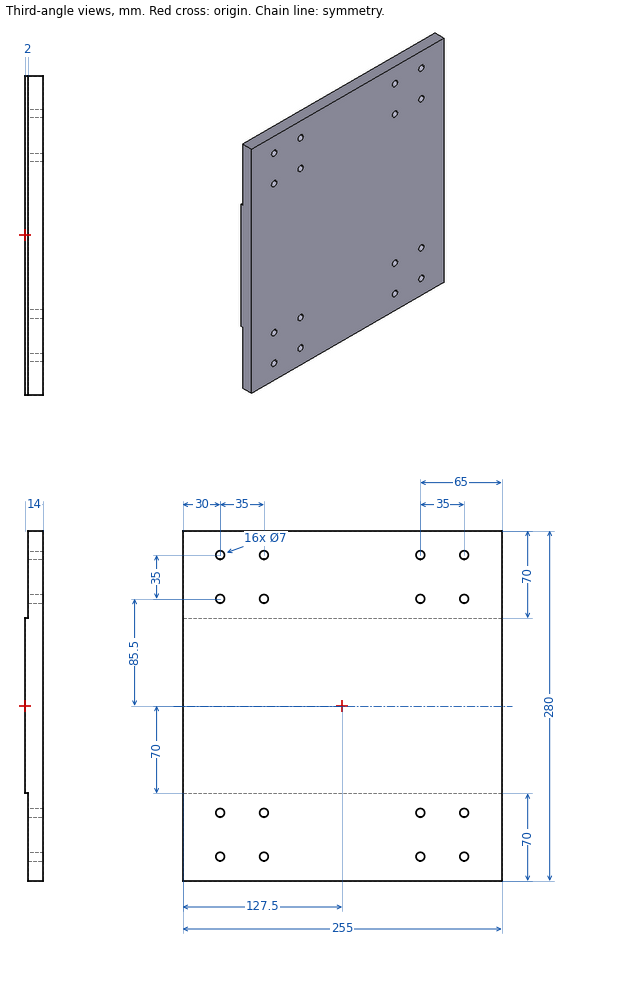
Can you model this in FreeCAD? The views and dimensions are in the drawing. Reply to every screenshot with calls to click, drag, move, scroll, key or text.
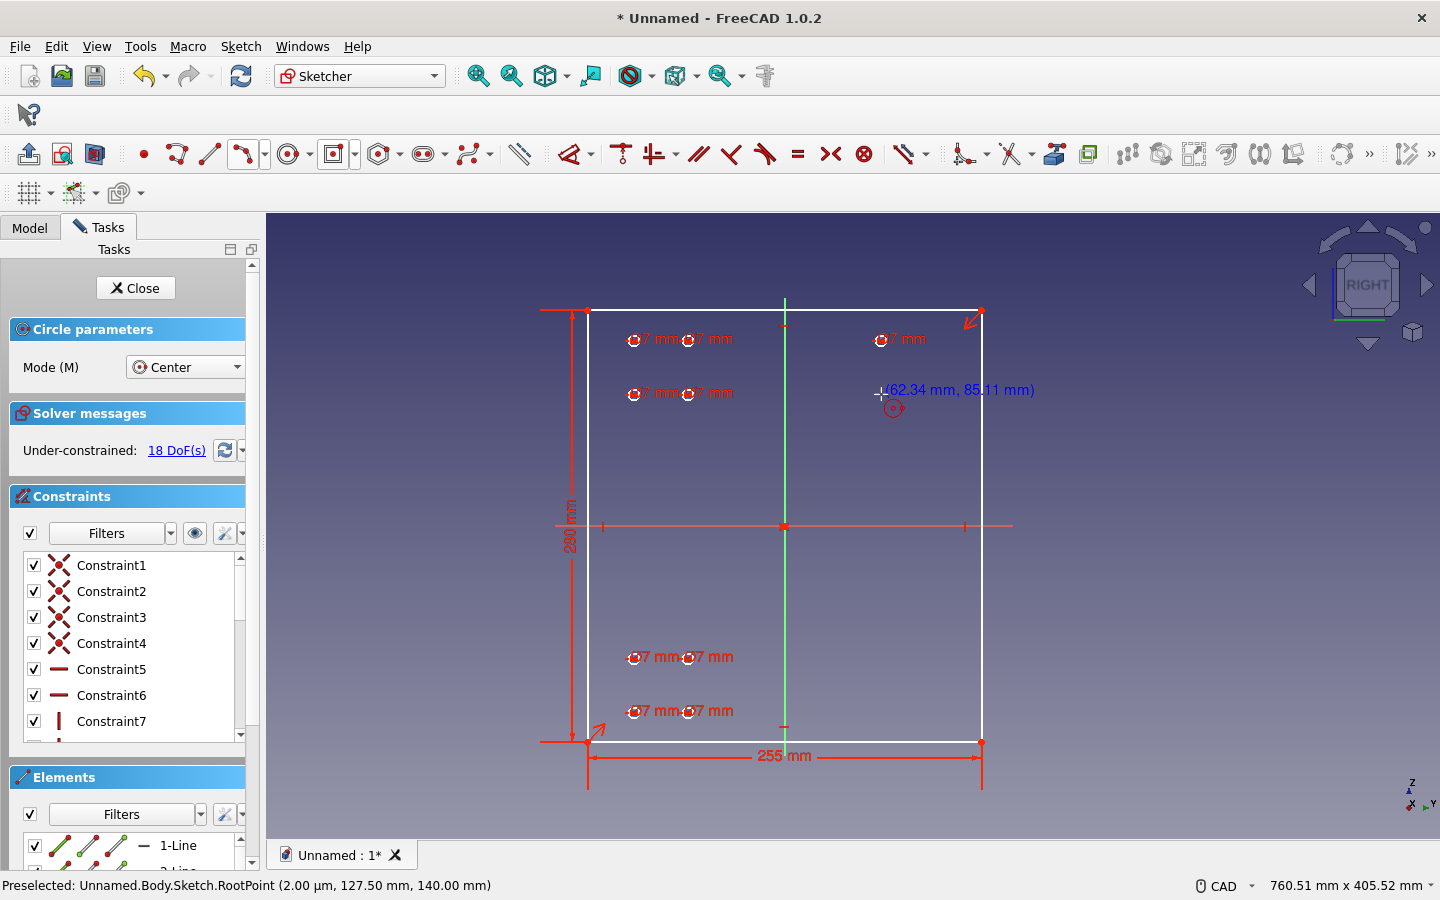
click(881, 394)
move(885, 391)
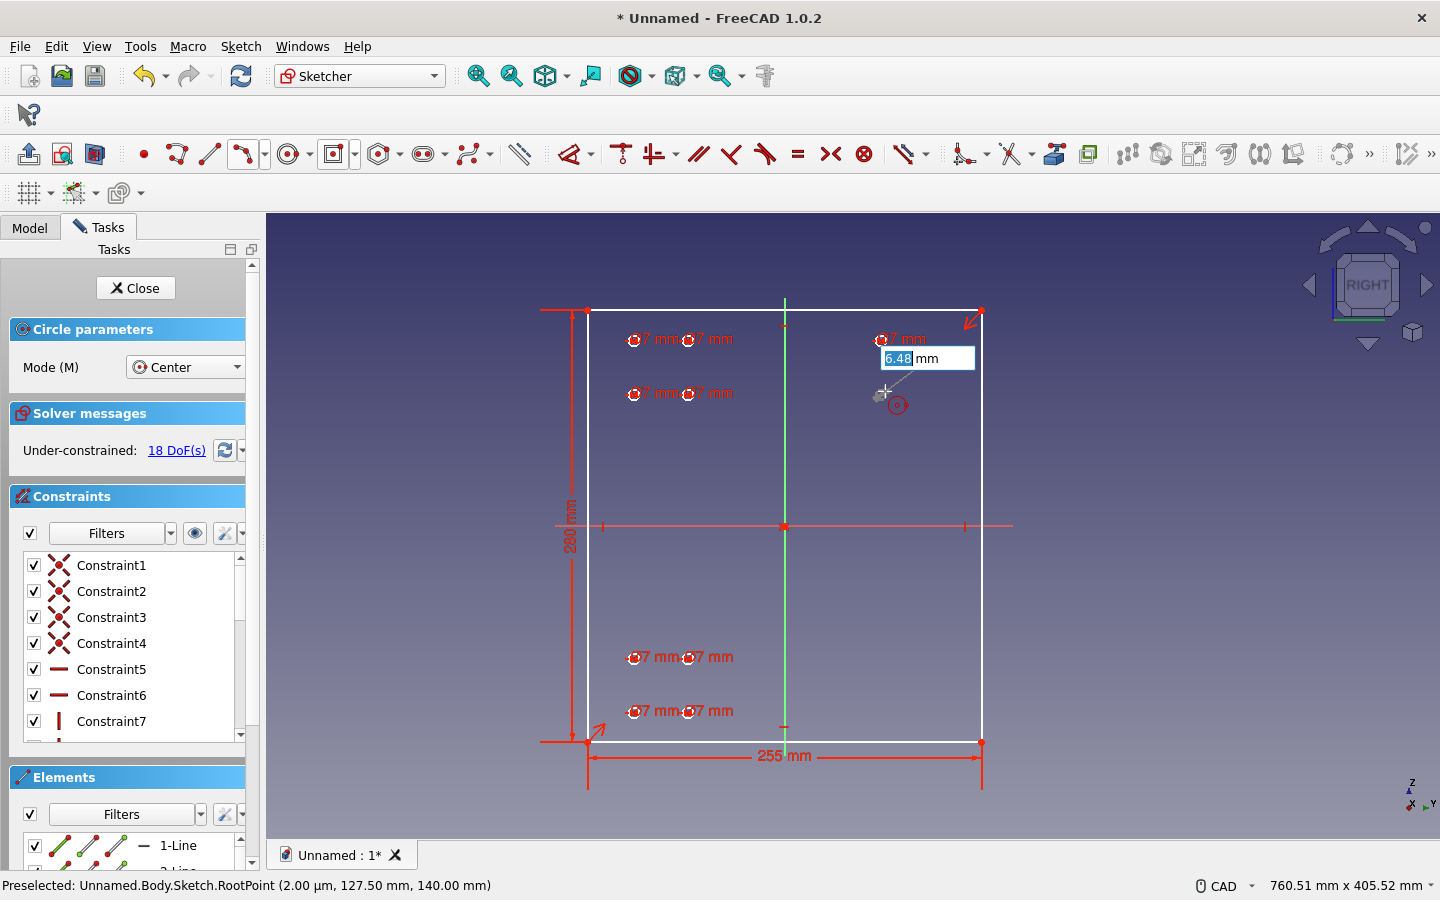
text(7)
key(Return)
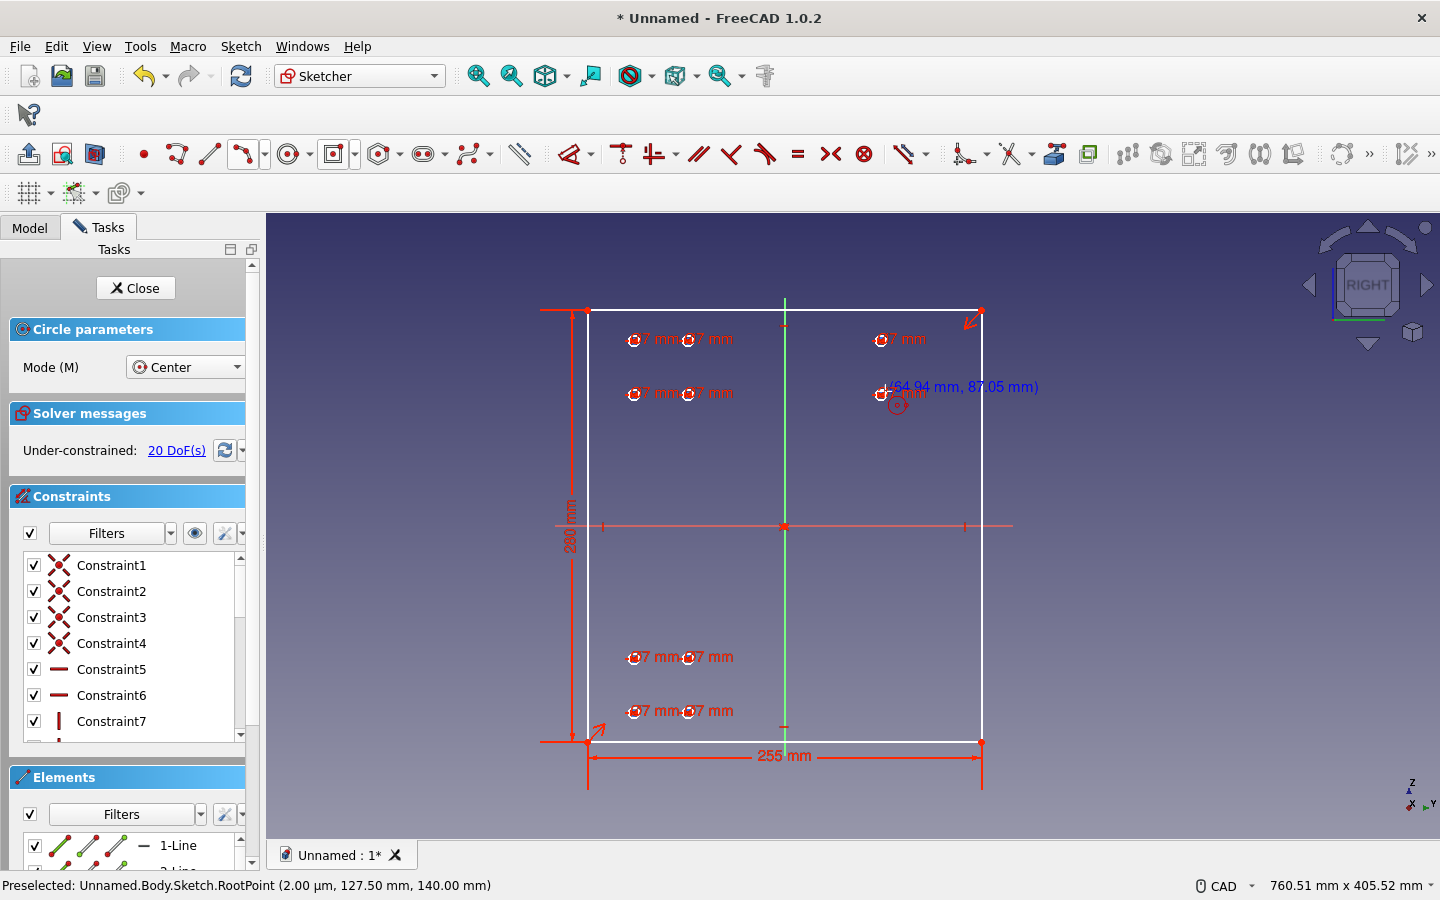
scroll(935, 340, up, 8)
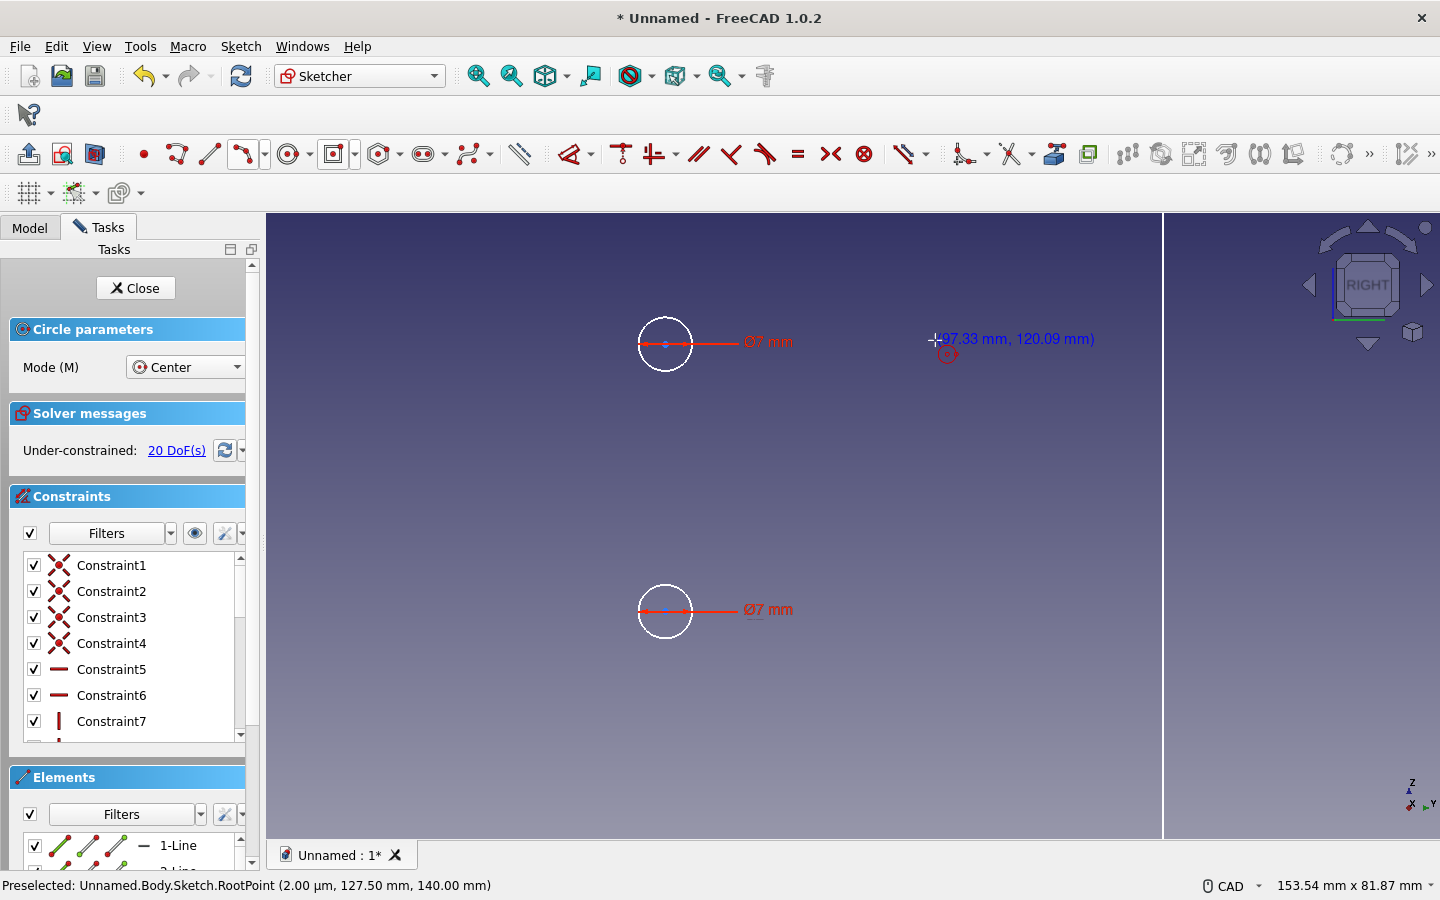
scroll(935, 340, down, 8)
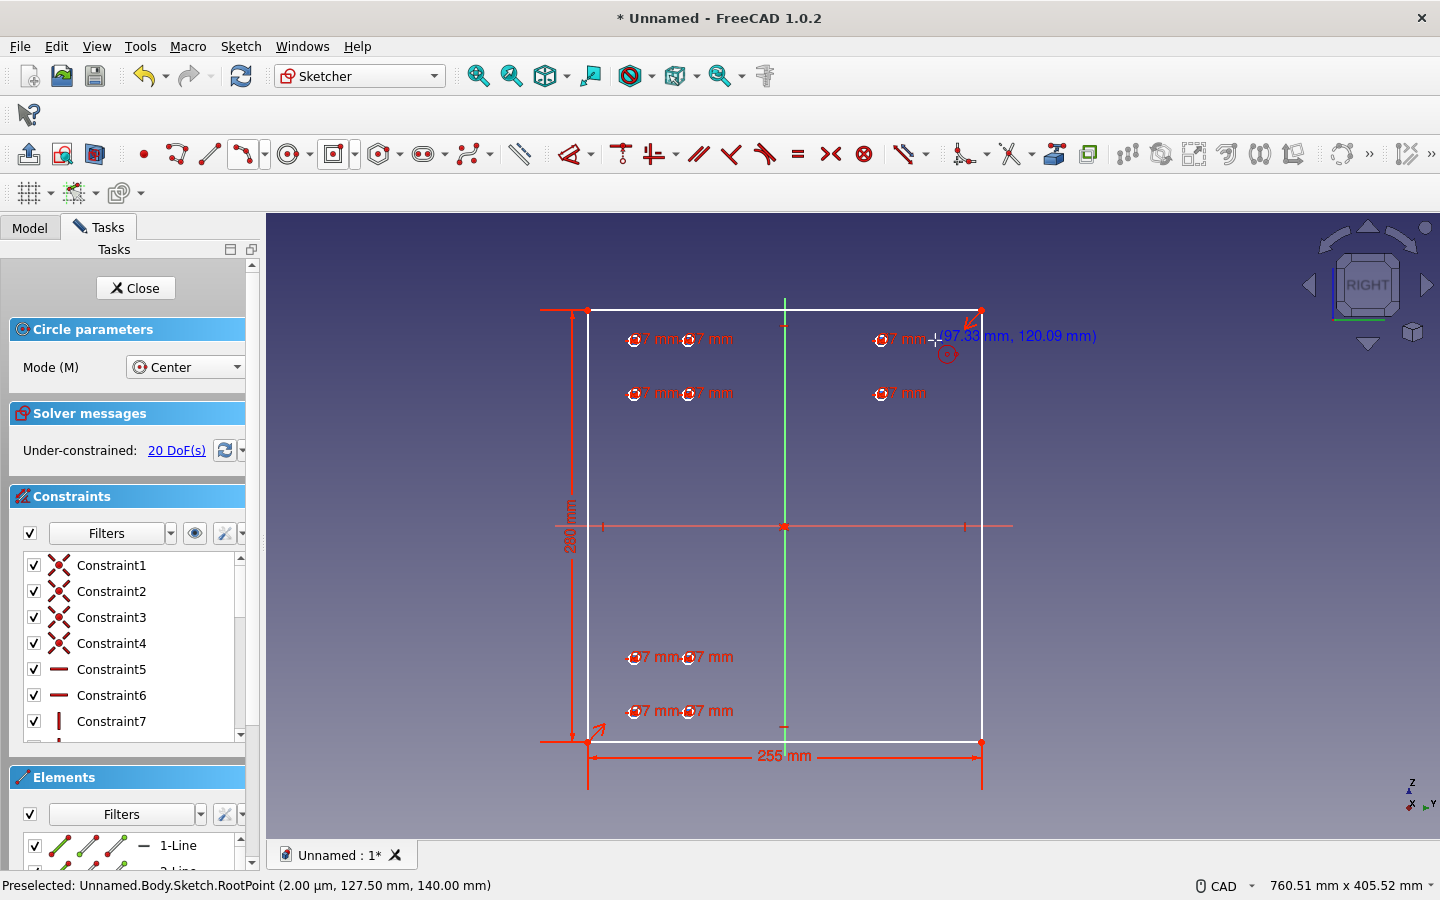
click(935, 340)
move(939, 337)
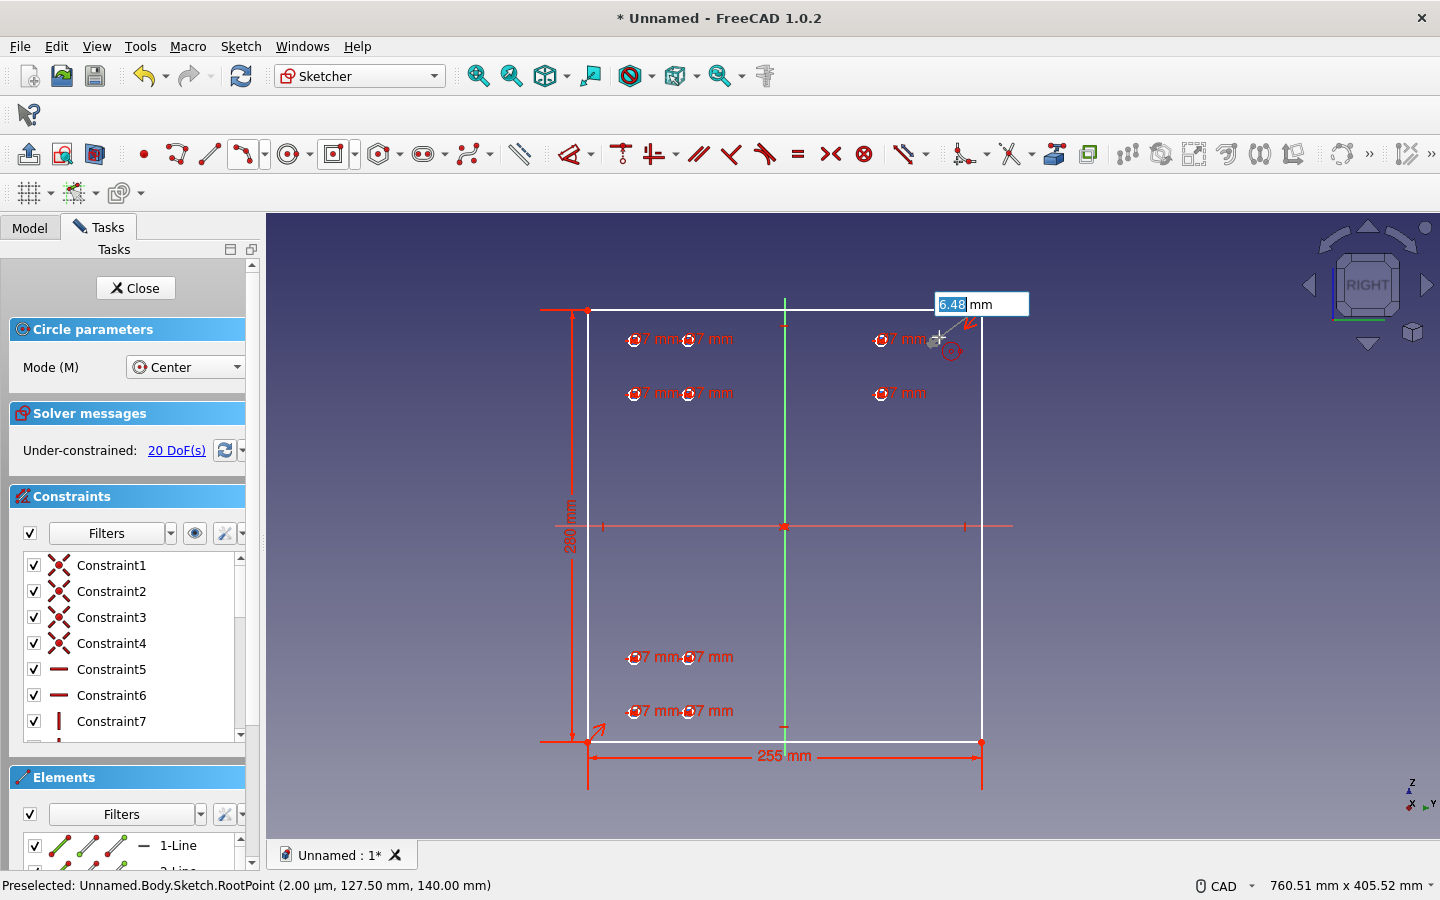
text(7)
key(Return)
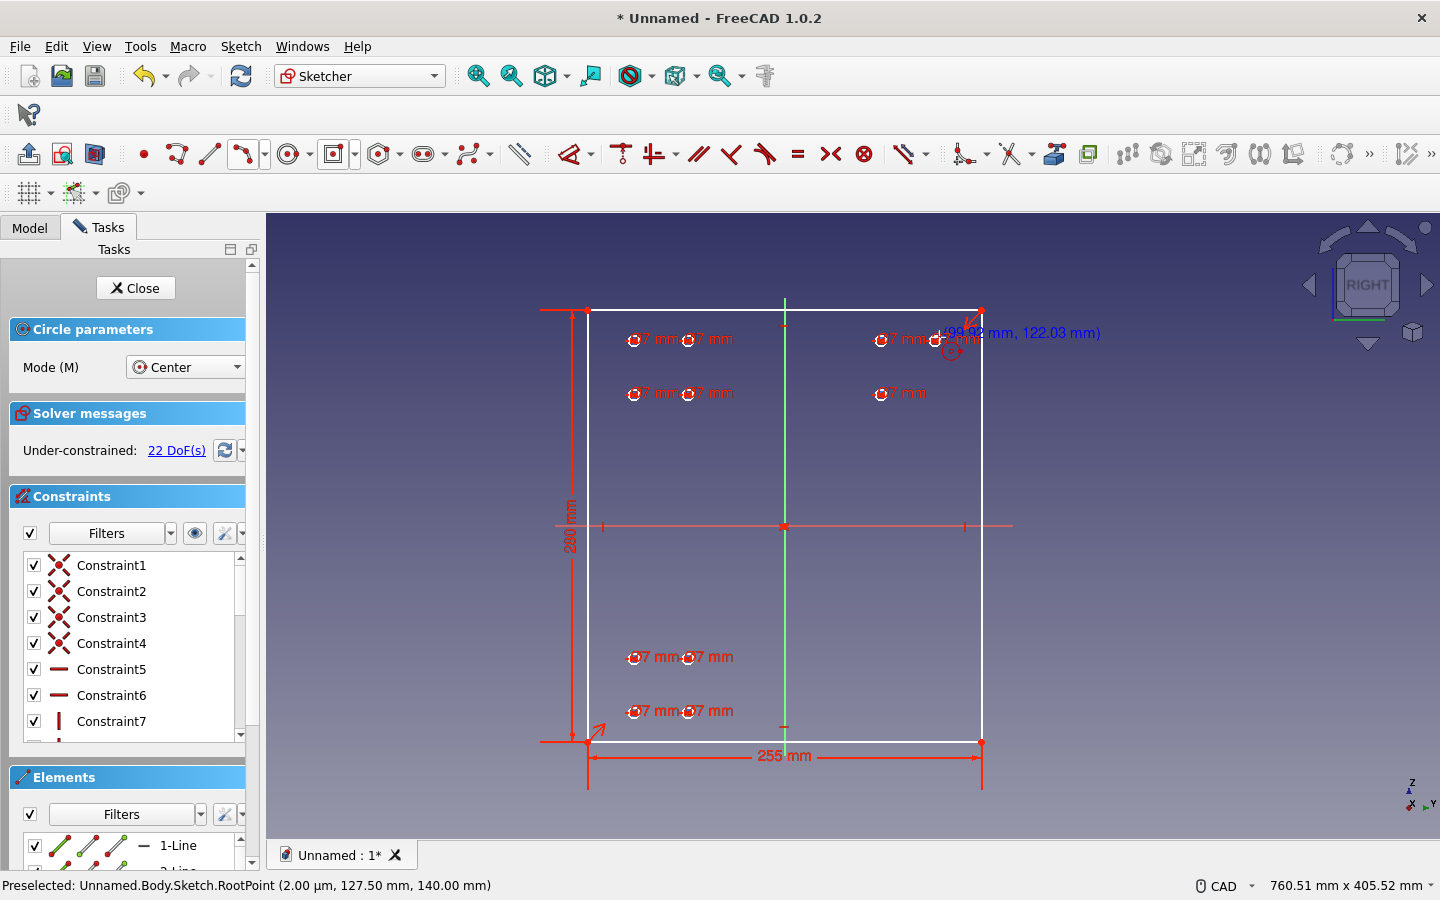
scroll(935, 394, up, 8)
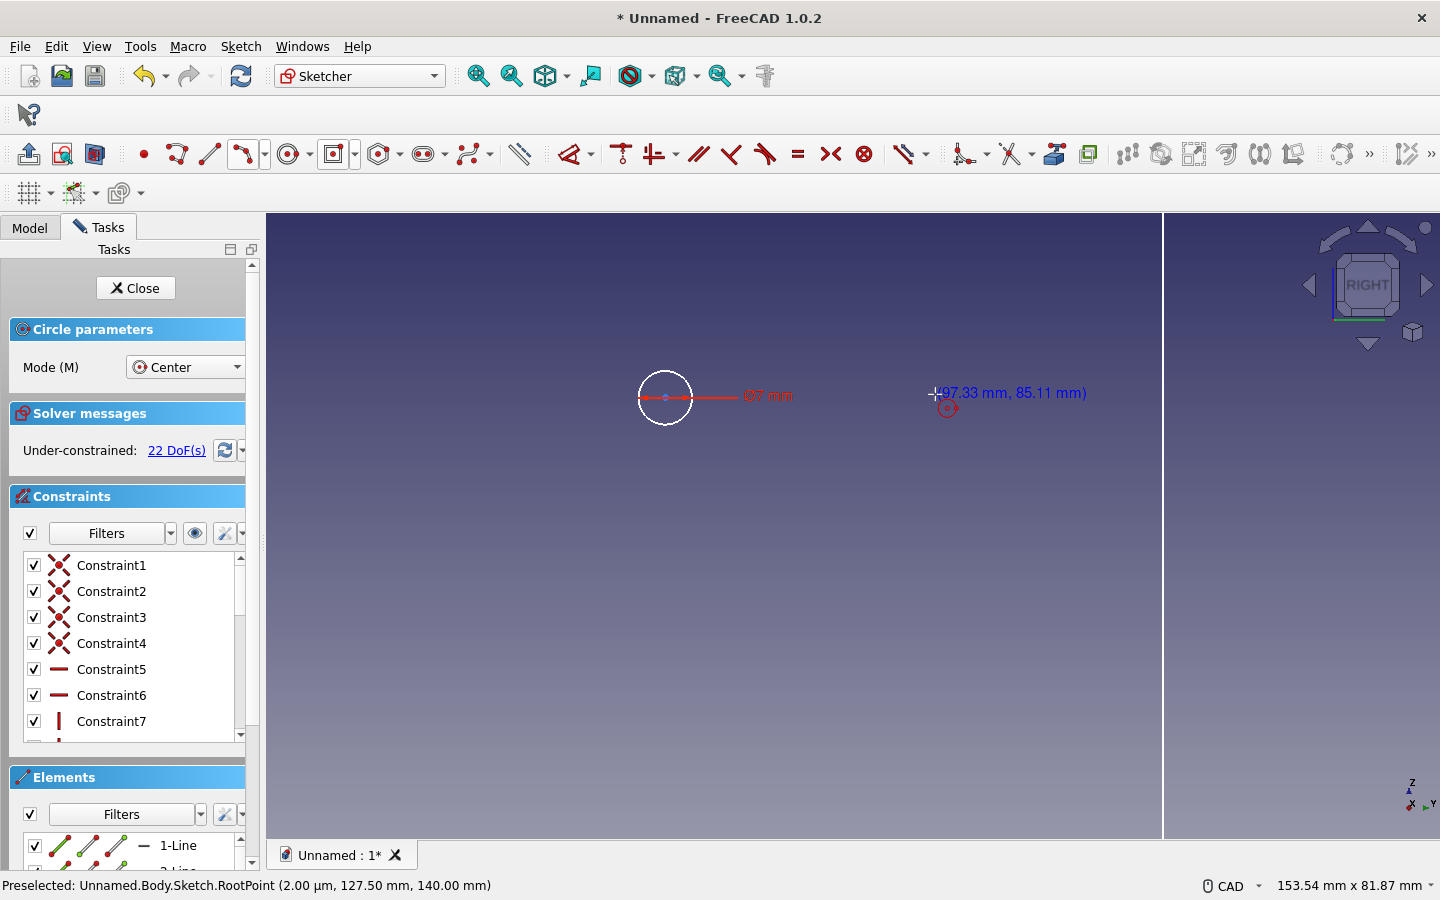
scroll(935, 394, down, 8)